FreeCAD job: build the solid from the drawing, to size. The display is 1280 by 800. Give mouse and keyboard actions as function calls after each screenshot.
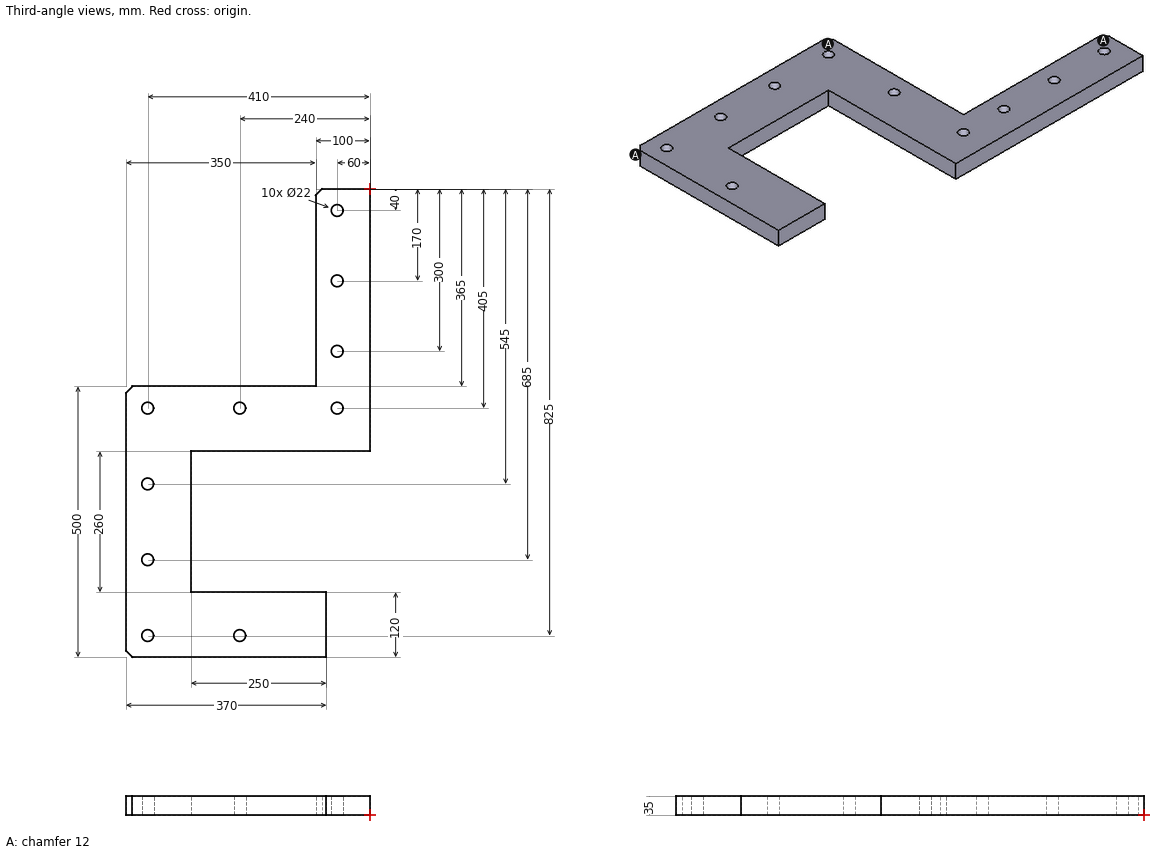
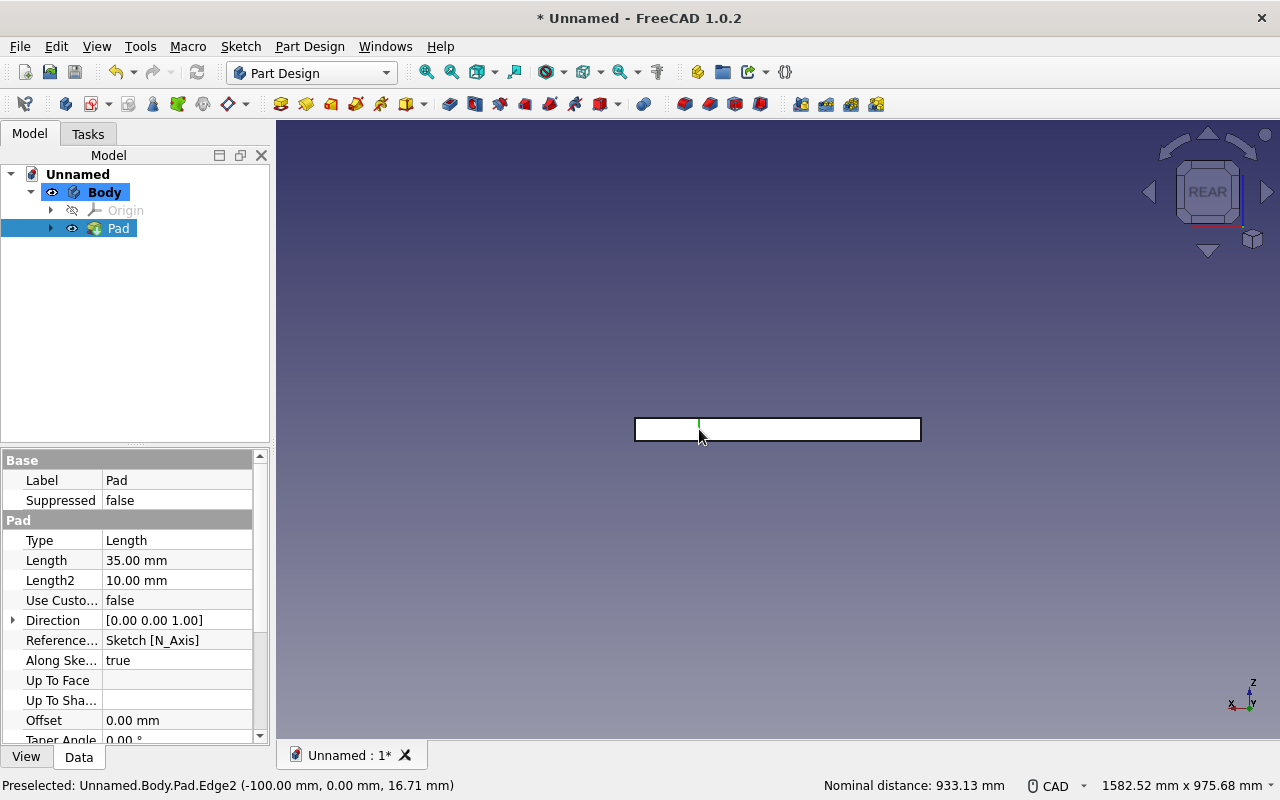
click(921, 429, ctrl)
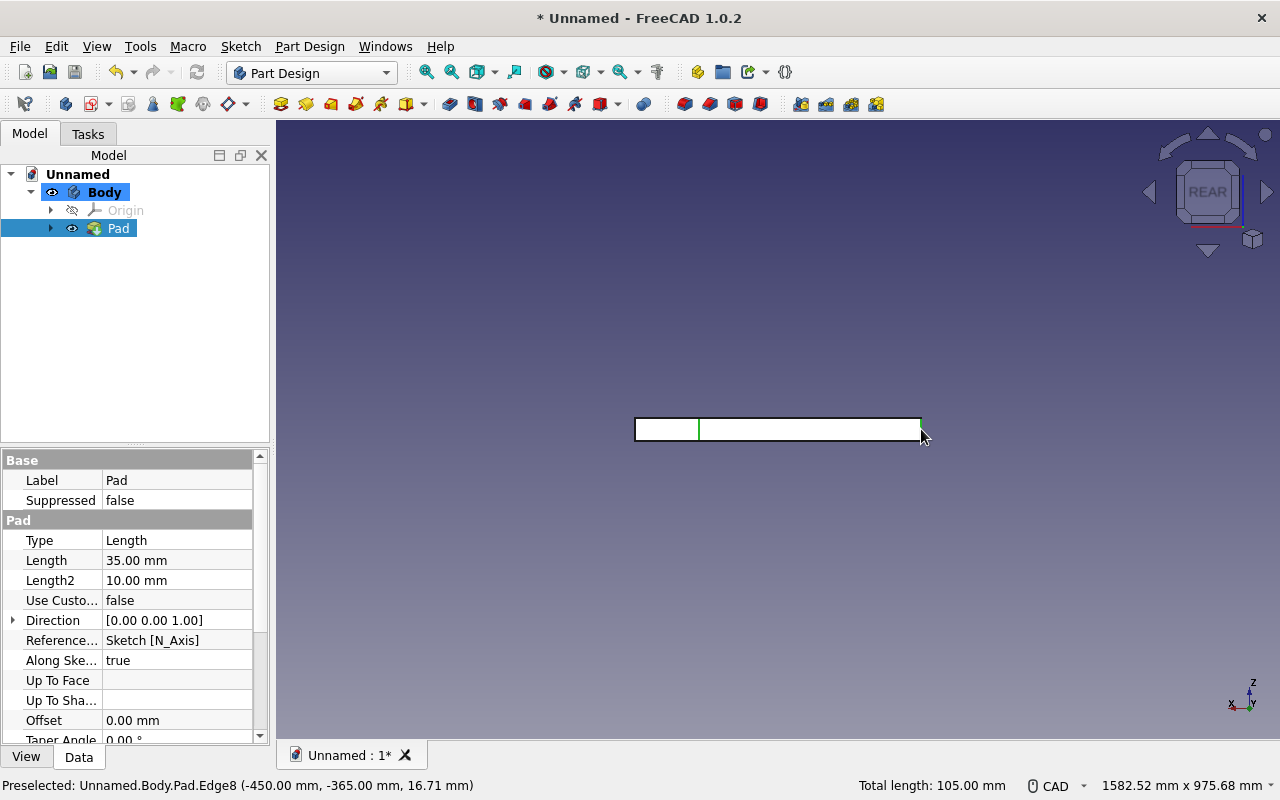
click(710, 104)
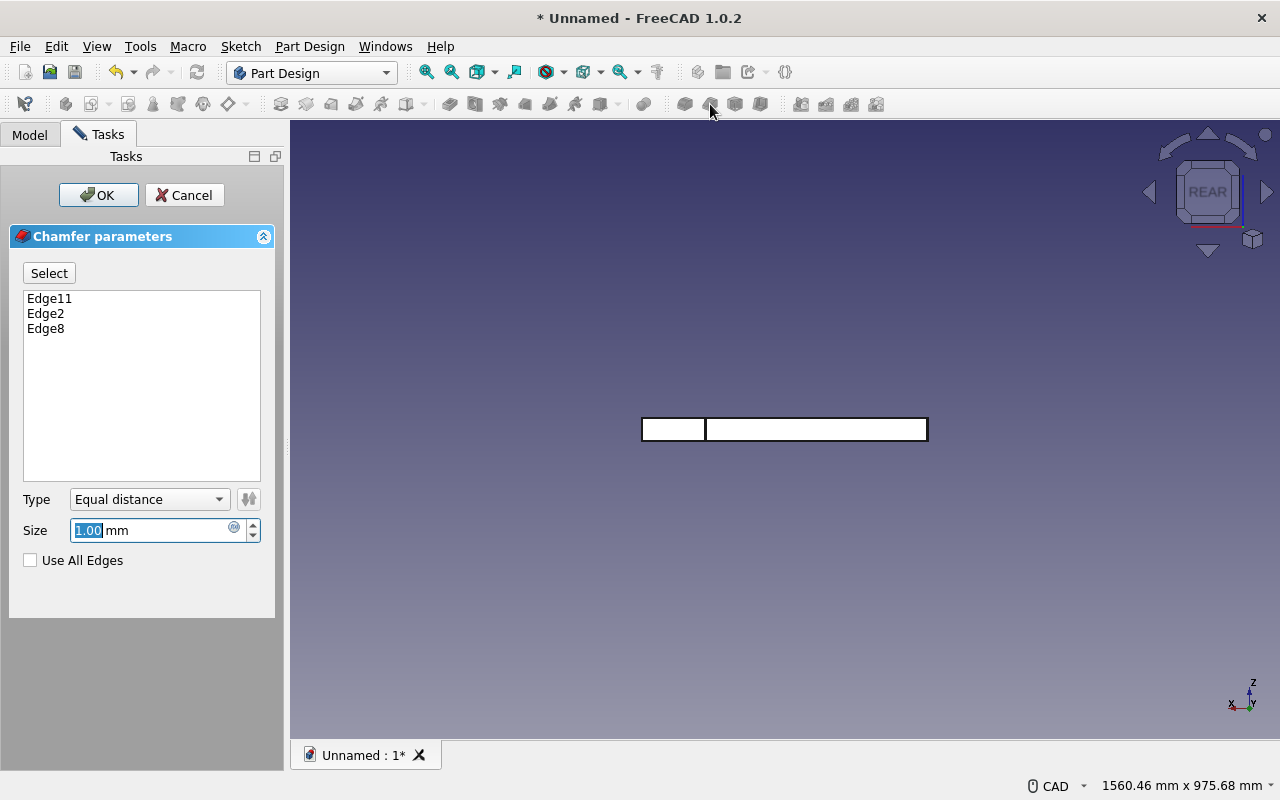
text(12)
key(Tab)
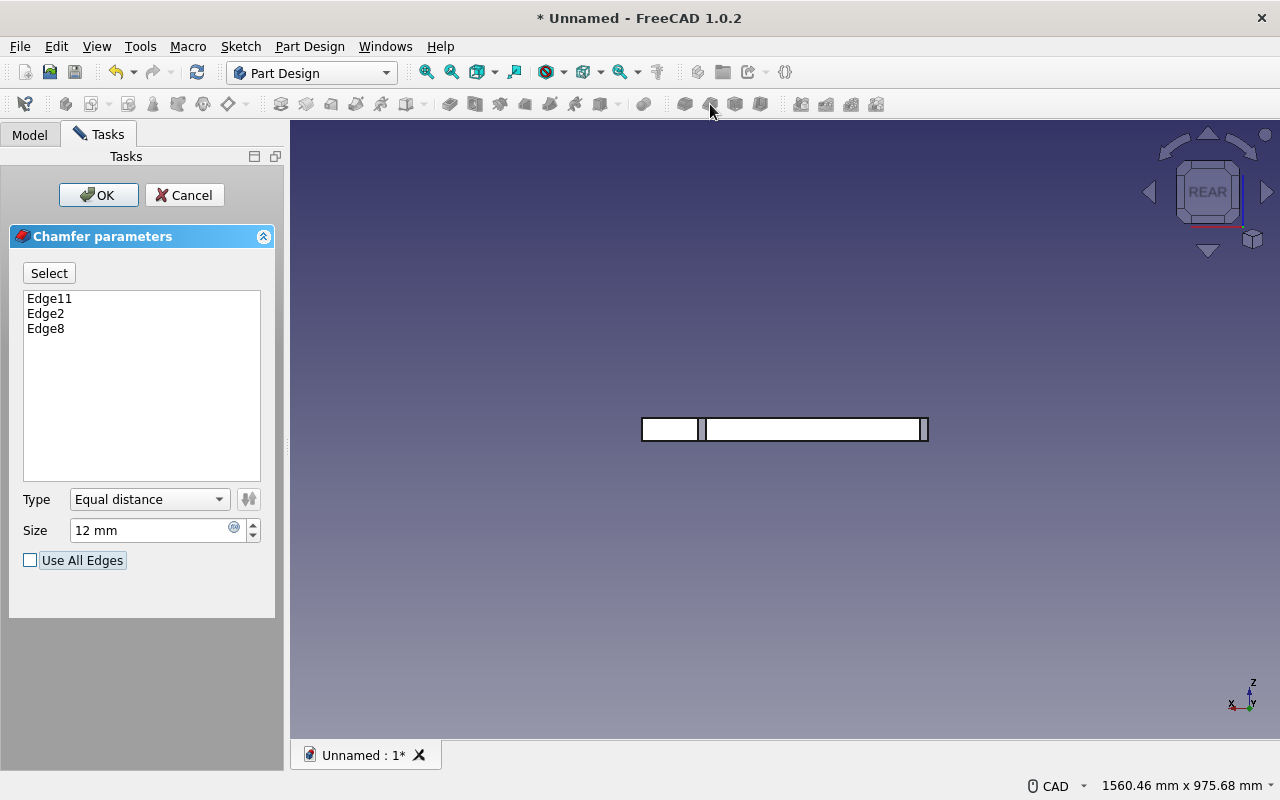
click(99, 195)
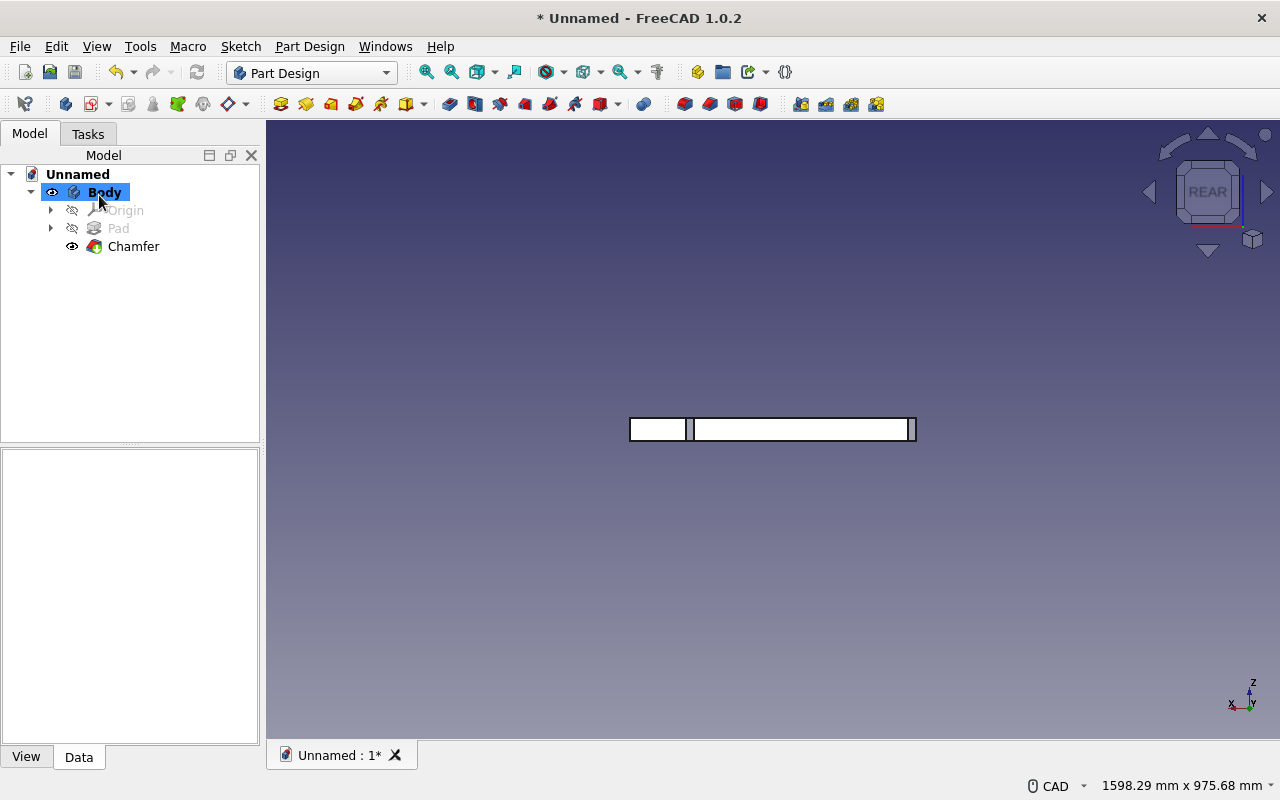
click(427, 72)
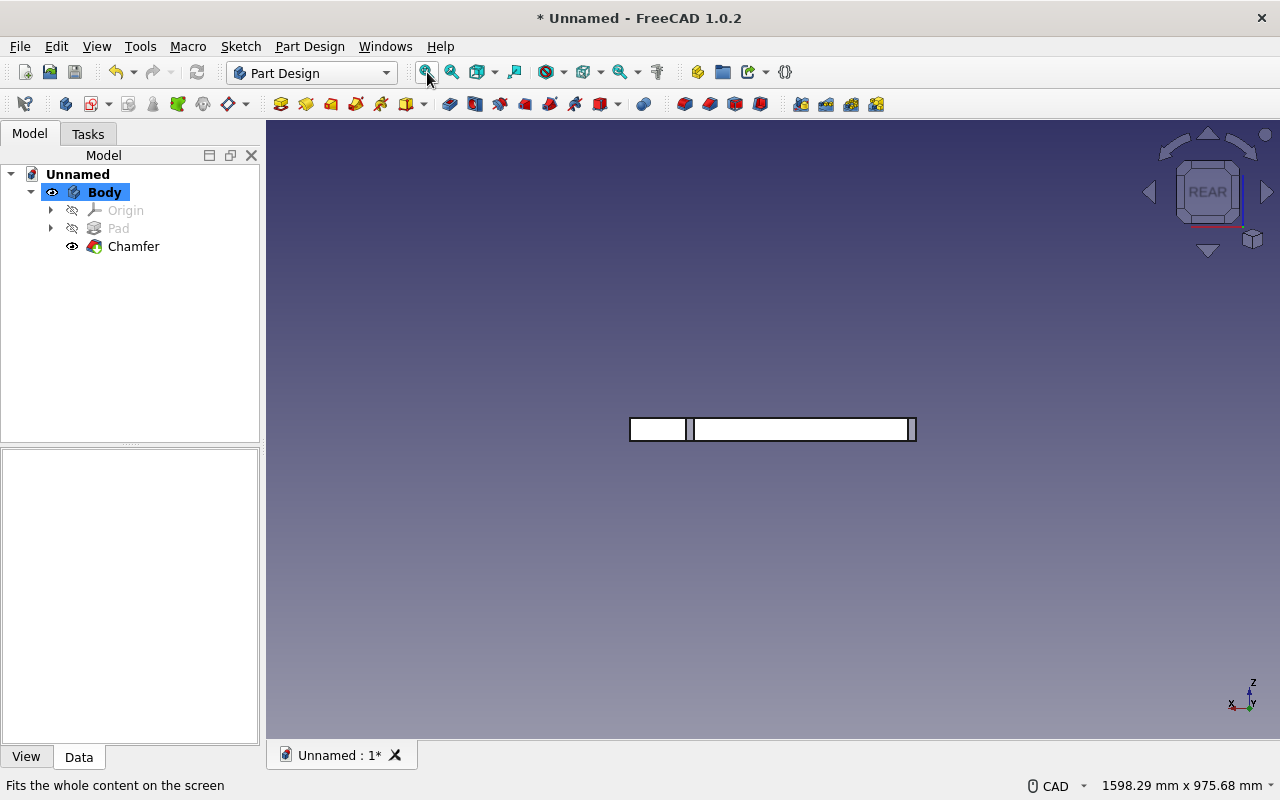
key(0)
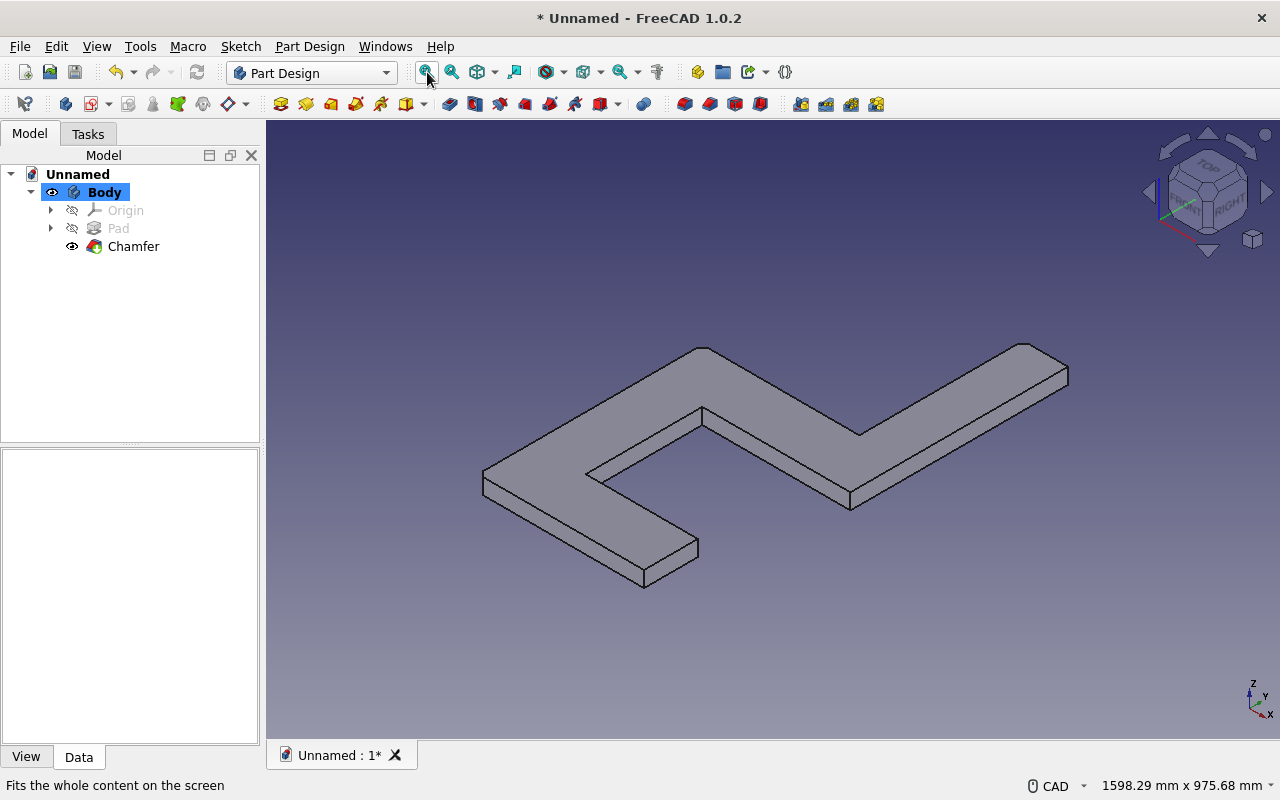
click(549, 482)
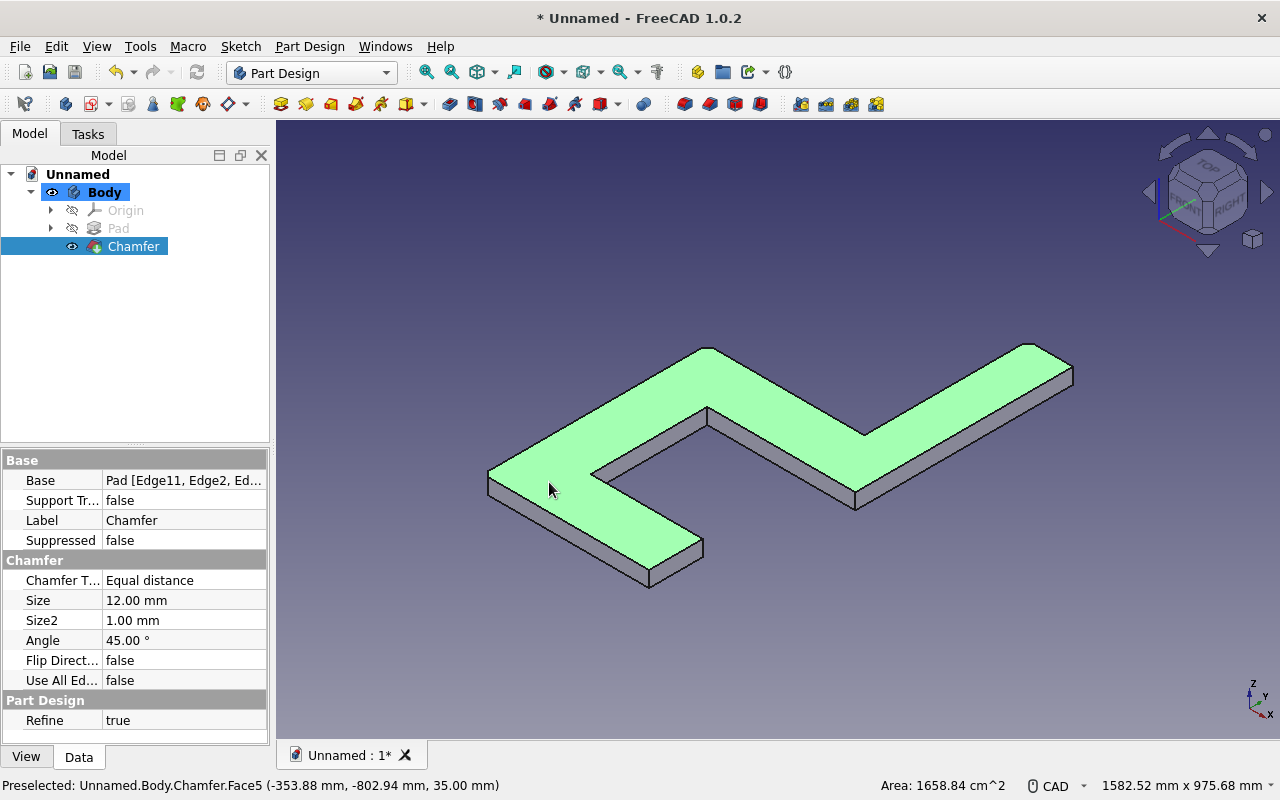
click(90, 104)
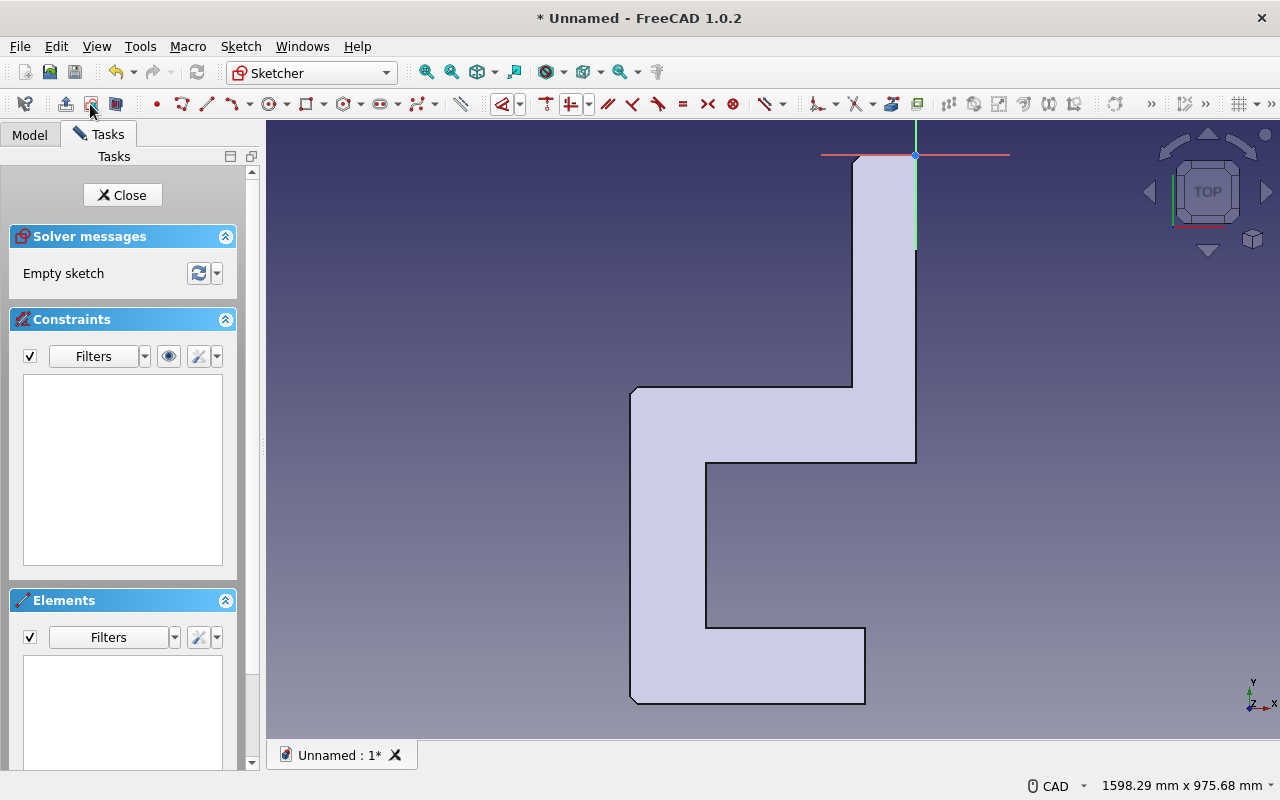
scroll(354, 471, down, 1)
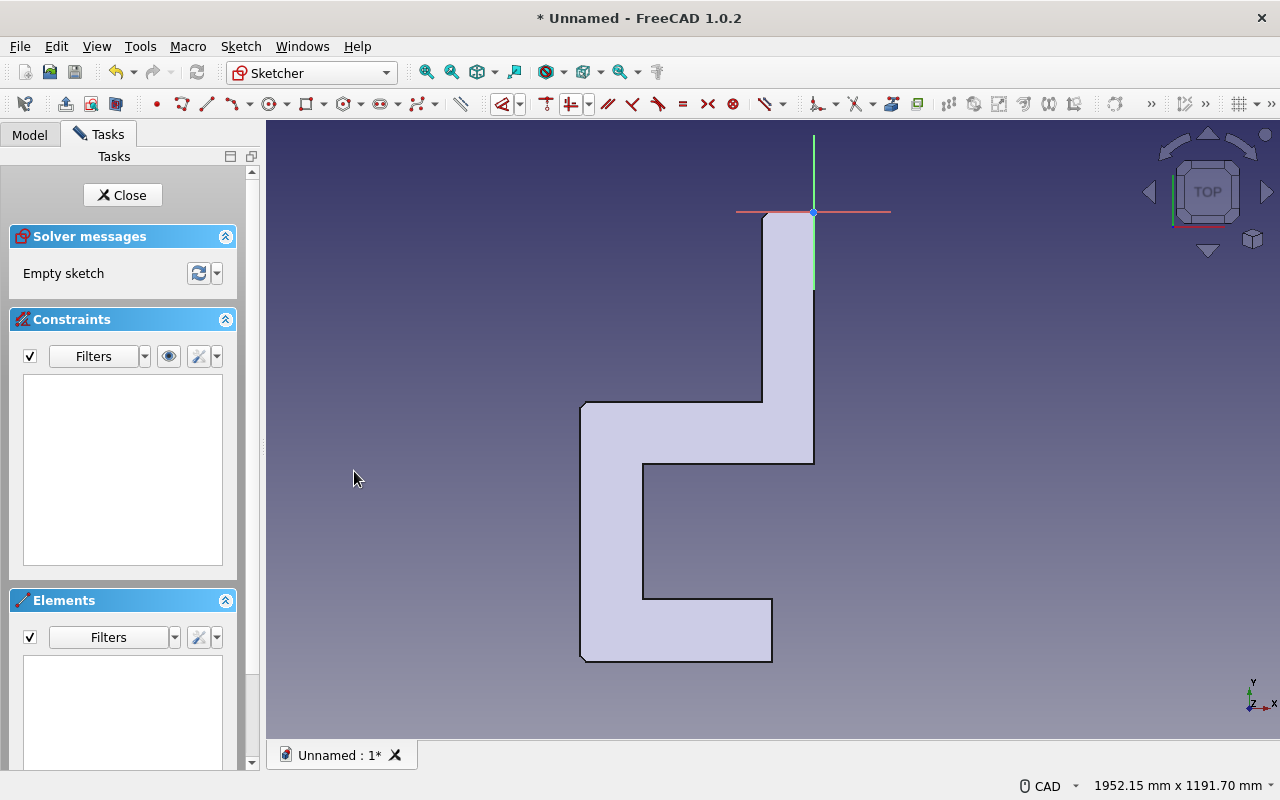
click(268, 104)